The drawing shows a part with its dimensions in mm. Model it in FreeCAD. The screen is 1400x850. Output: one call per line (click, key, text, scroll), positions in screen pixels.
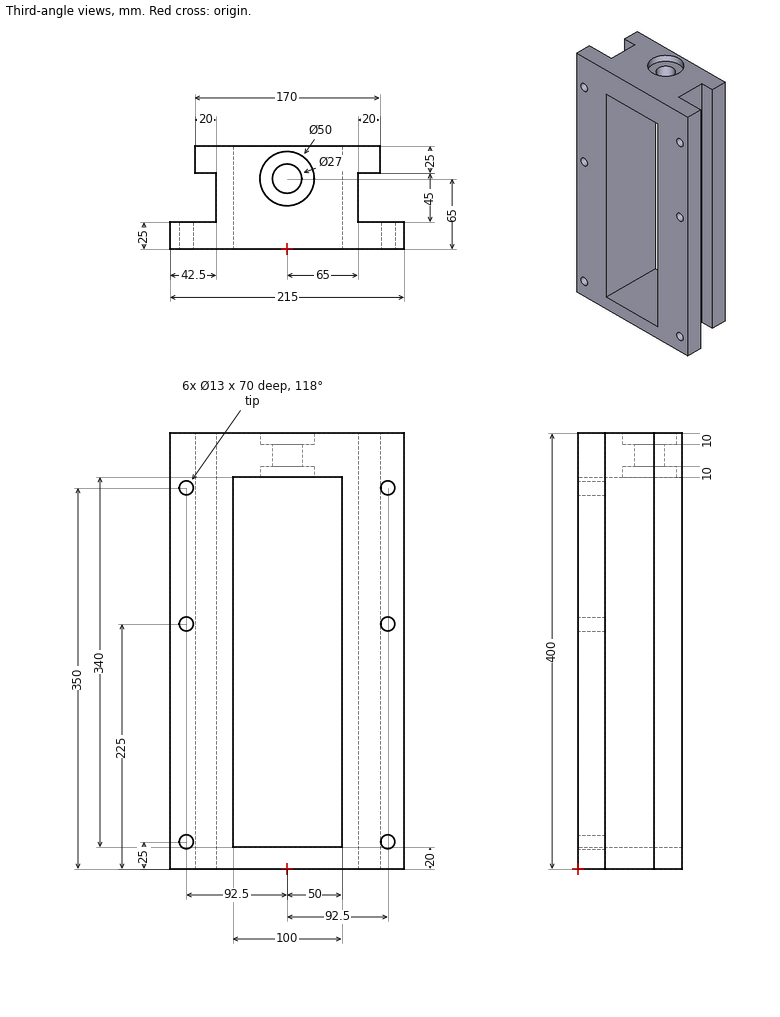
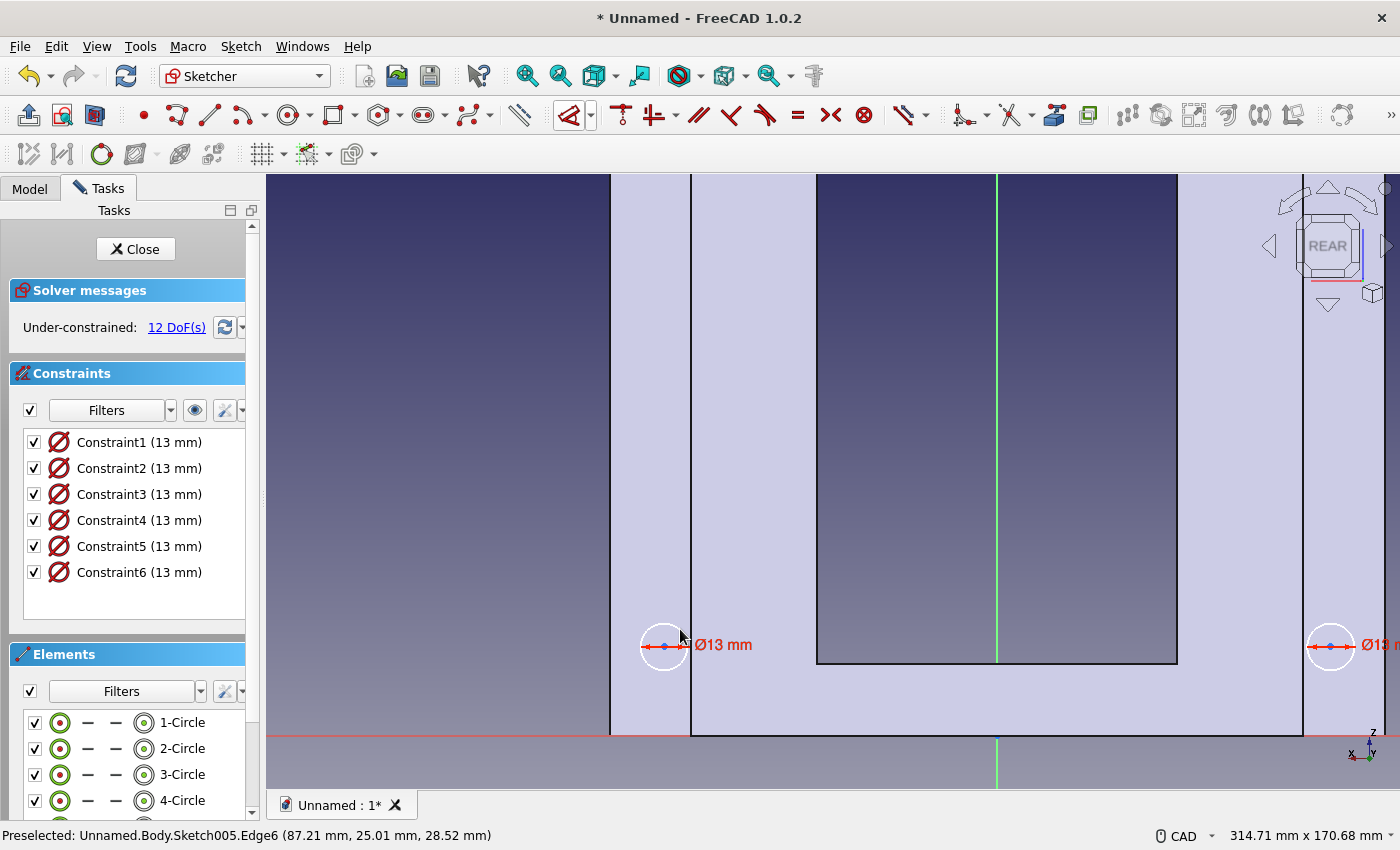
scroll(664, 649, down, 6)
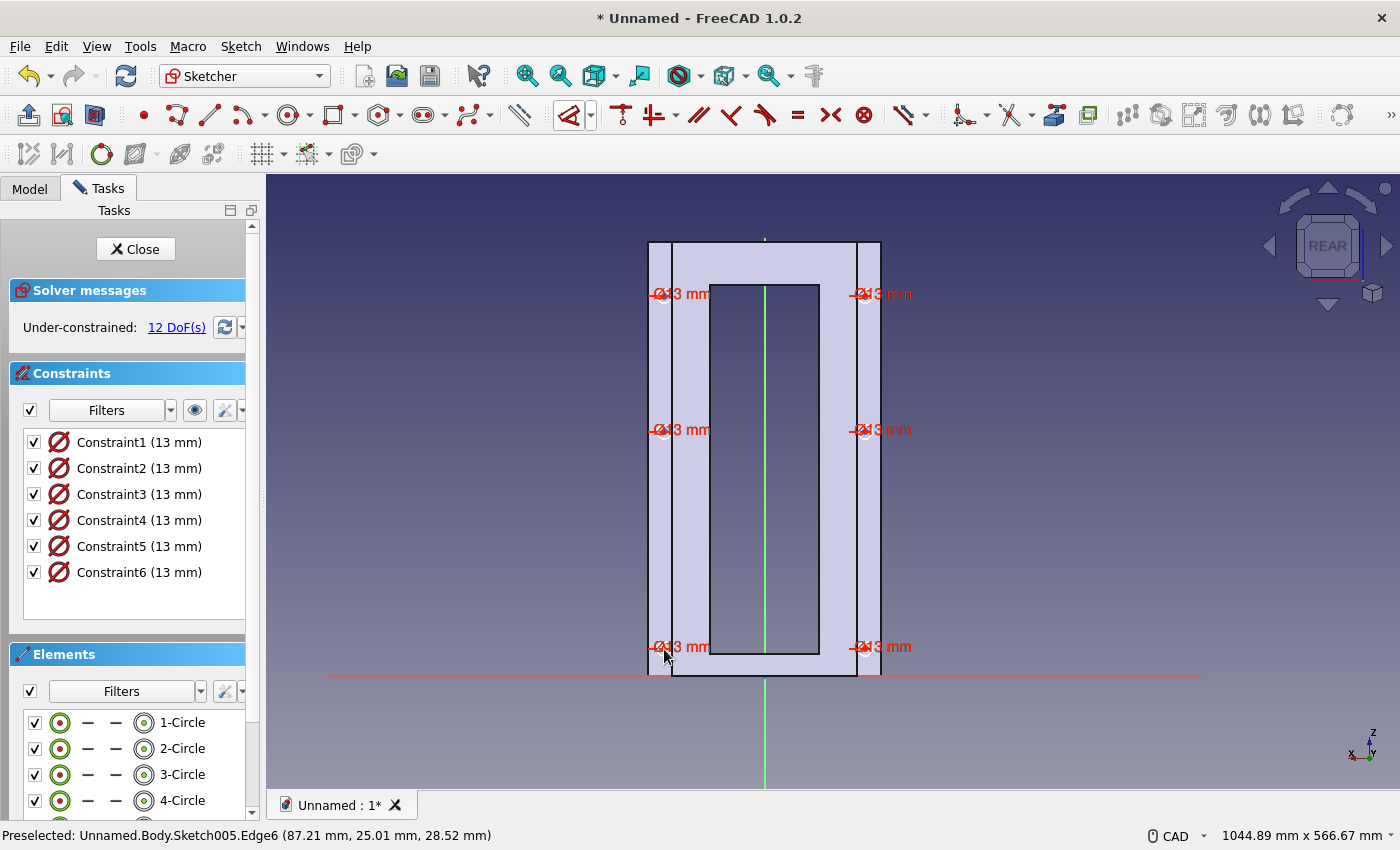
click(865, 296)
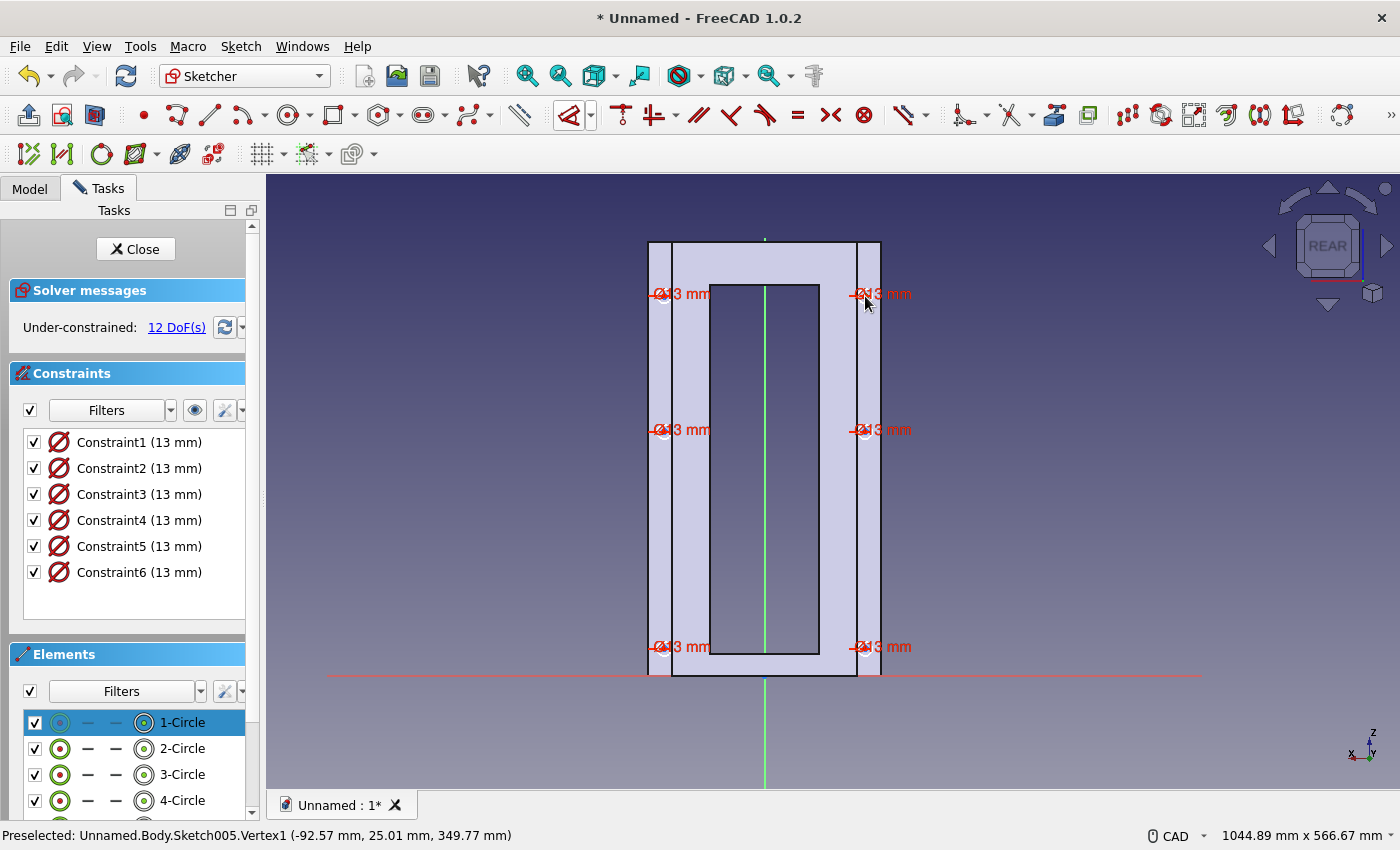
click(664, 296)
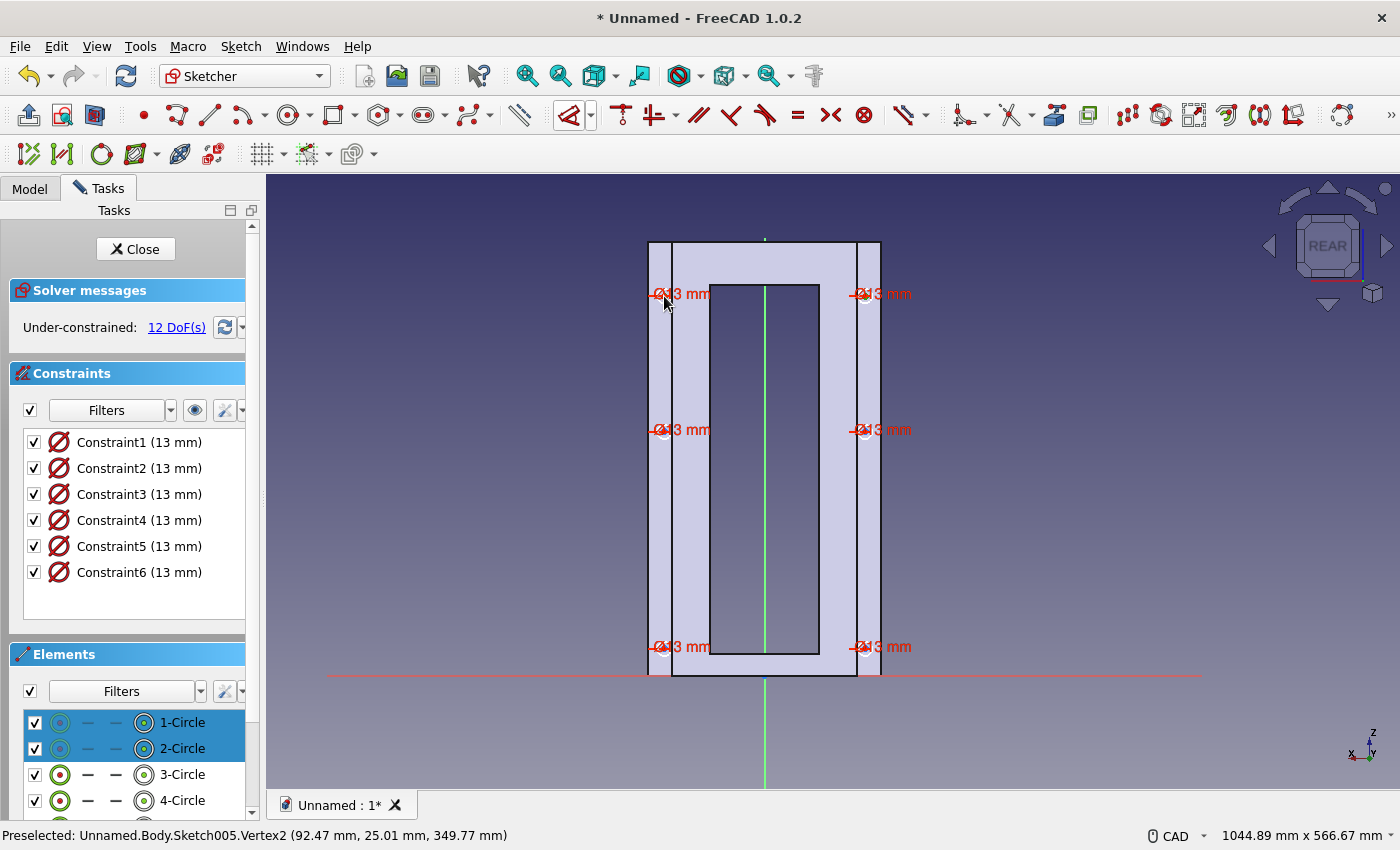
key(h)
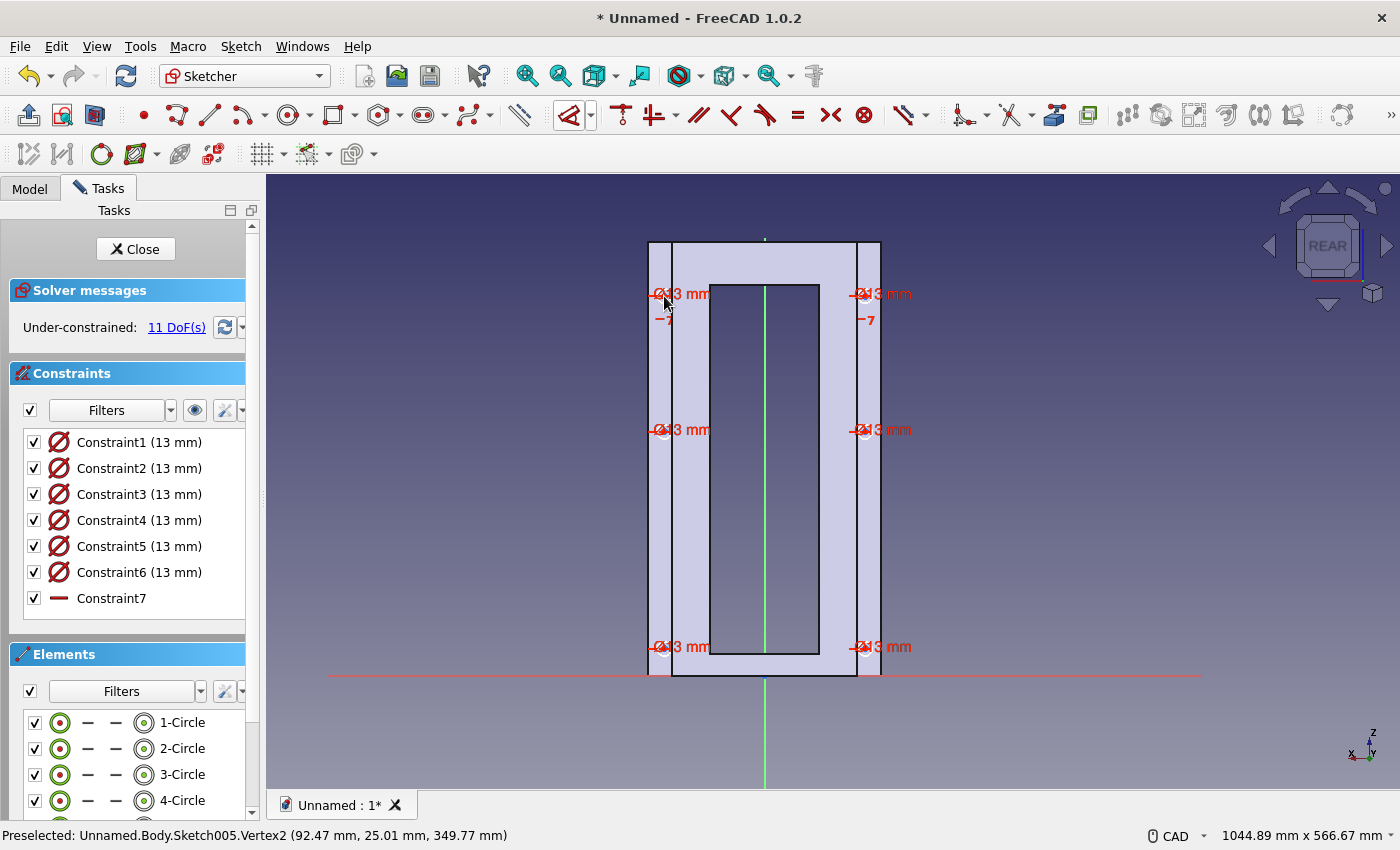
click(865, 296)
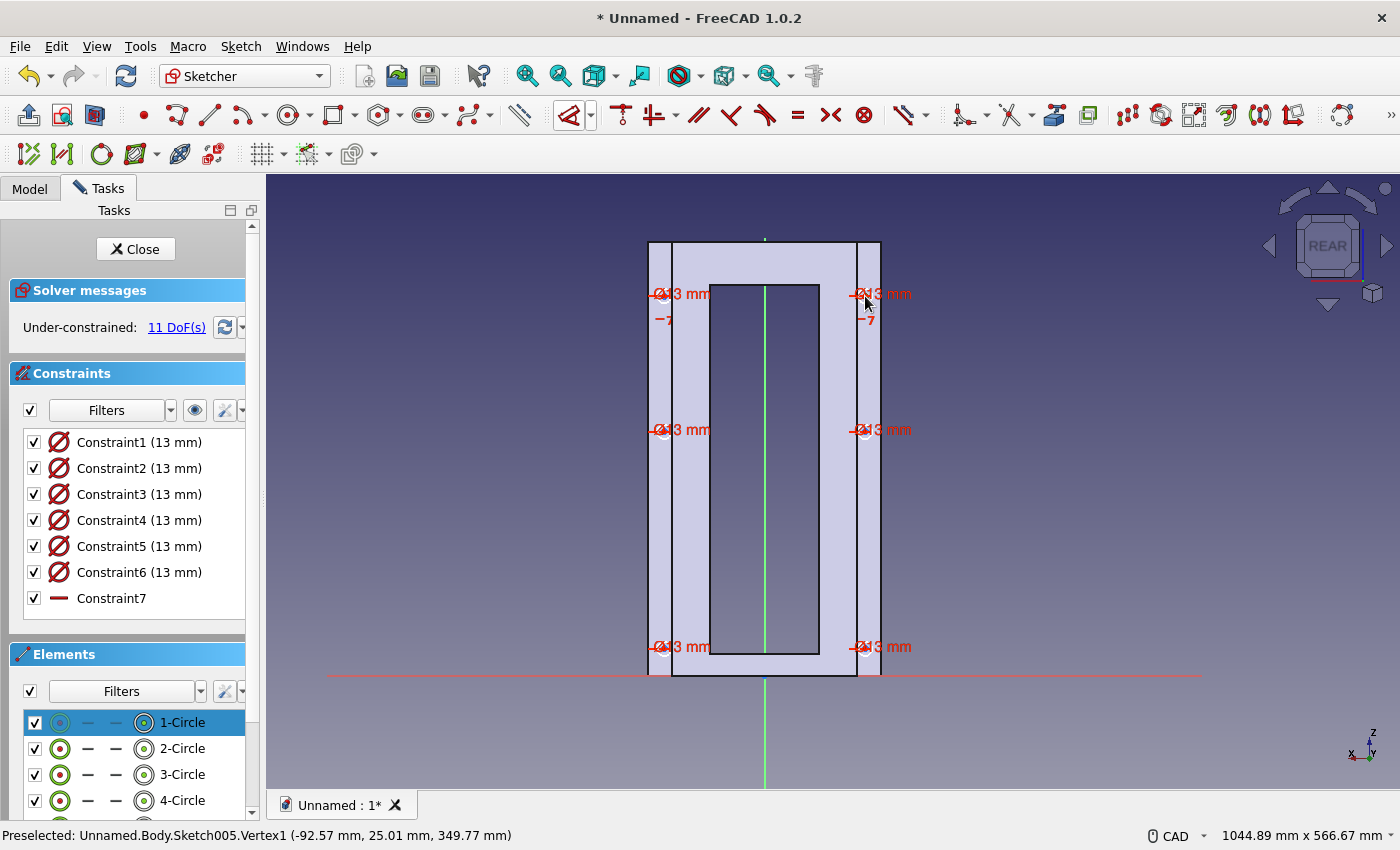
click(865, 432)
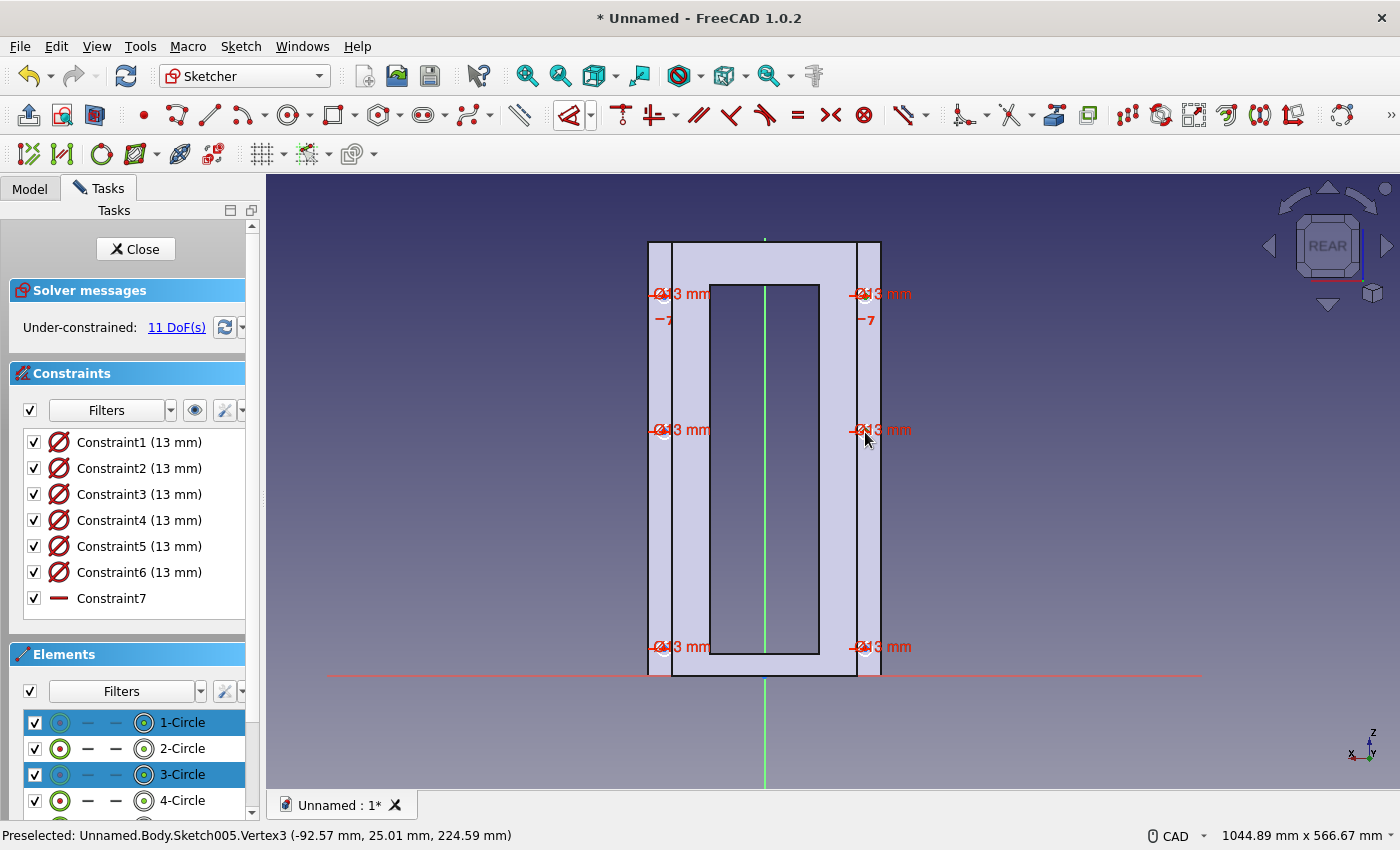
key(v)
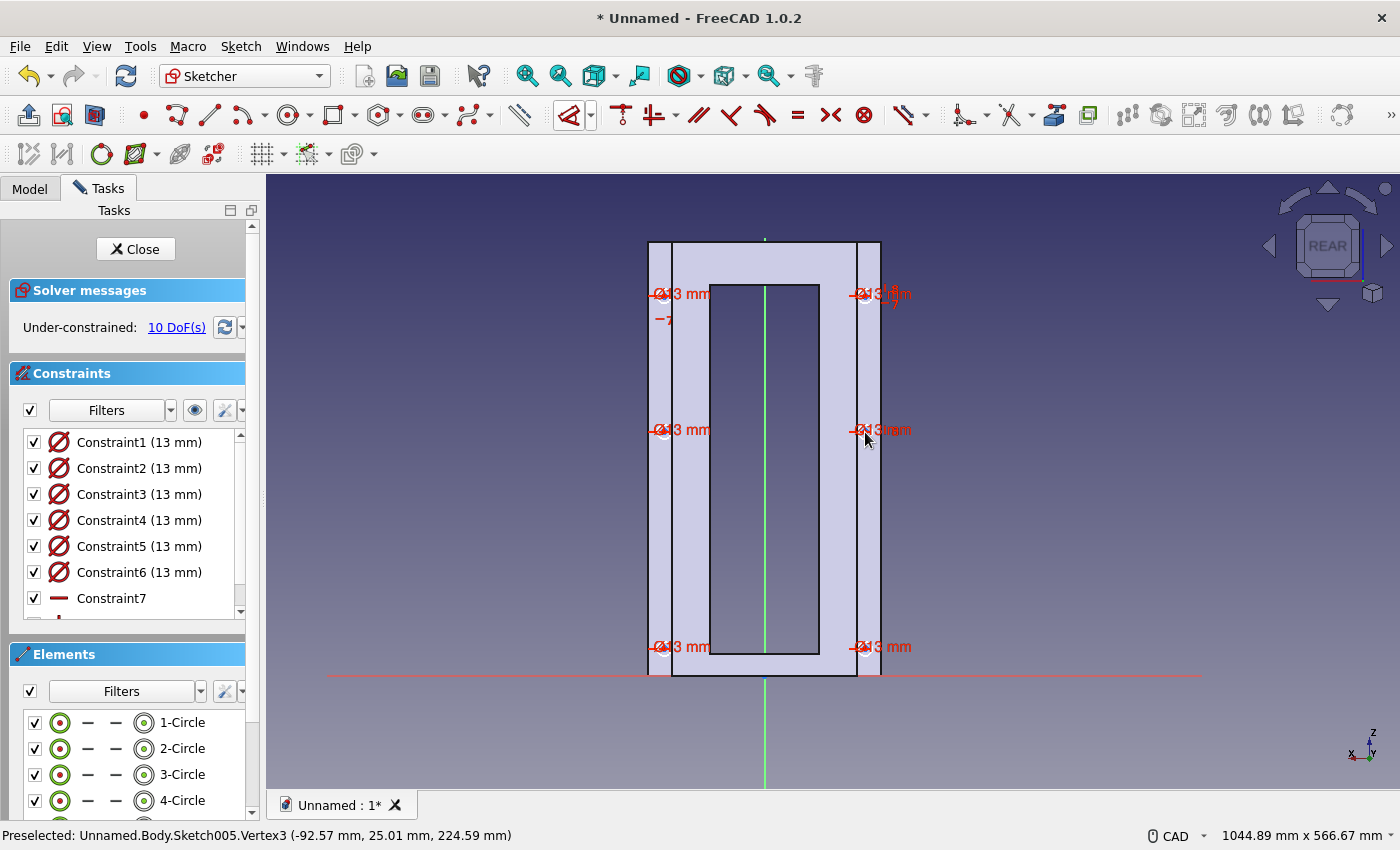
click(664, 296)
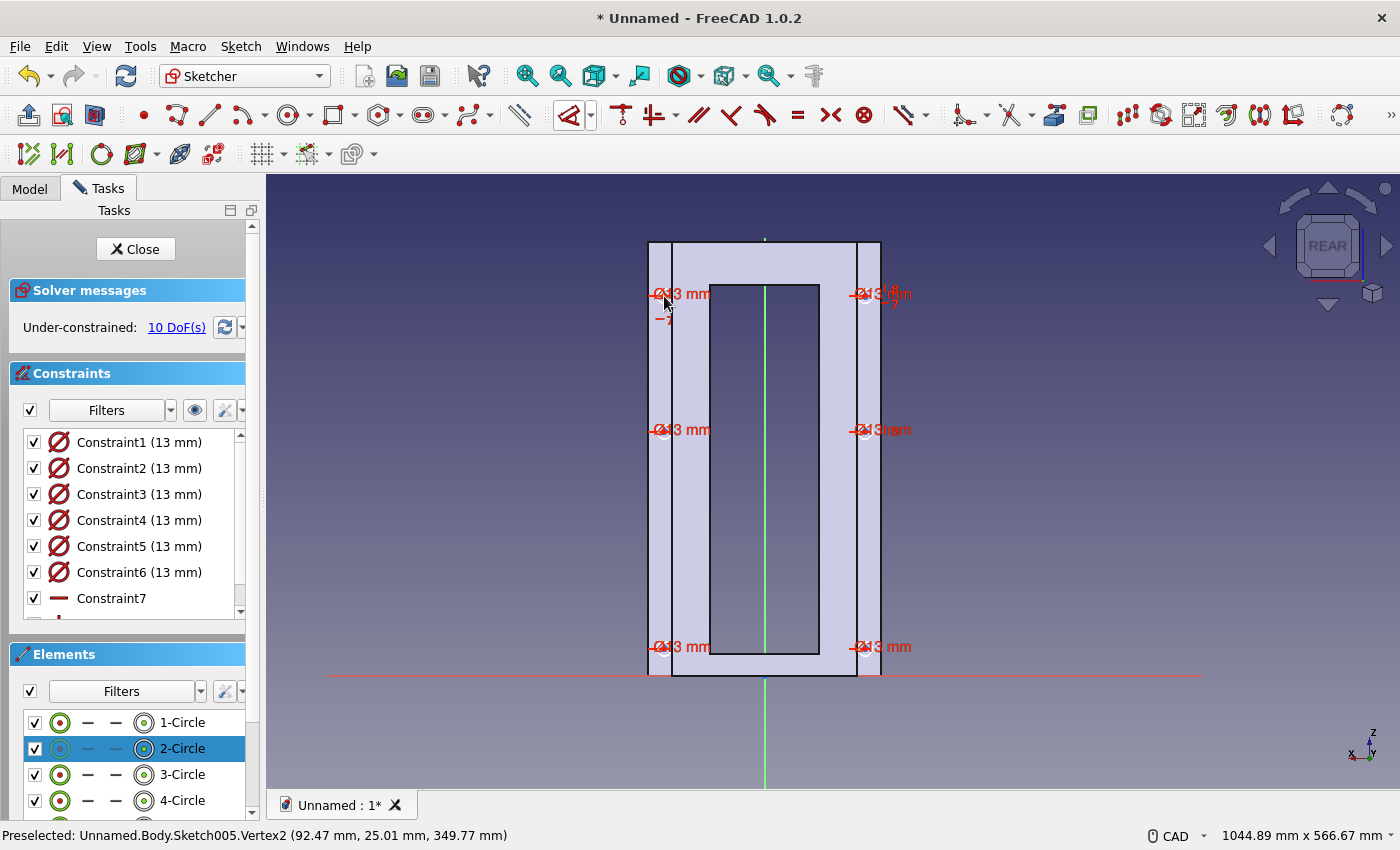
click(664, 432)